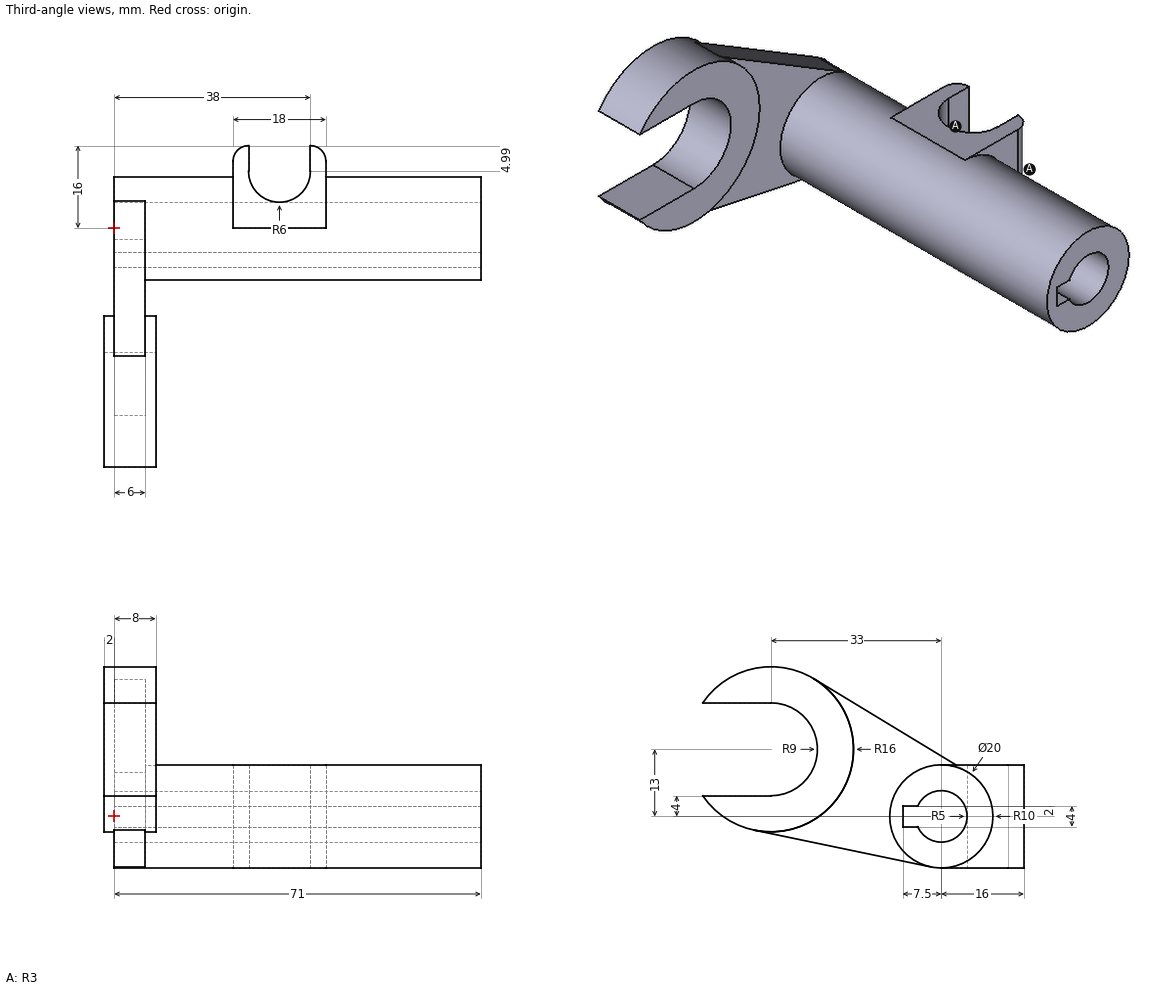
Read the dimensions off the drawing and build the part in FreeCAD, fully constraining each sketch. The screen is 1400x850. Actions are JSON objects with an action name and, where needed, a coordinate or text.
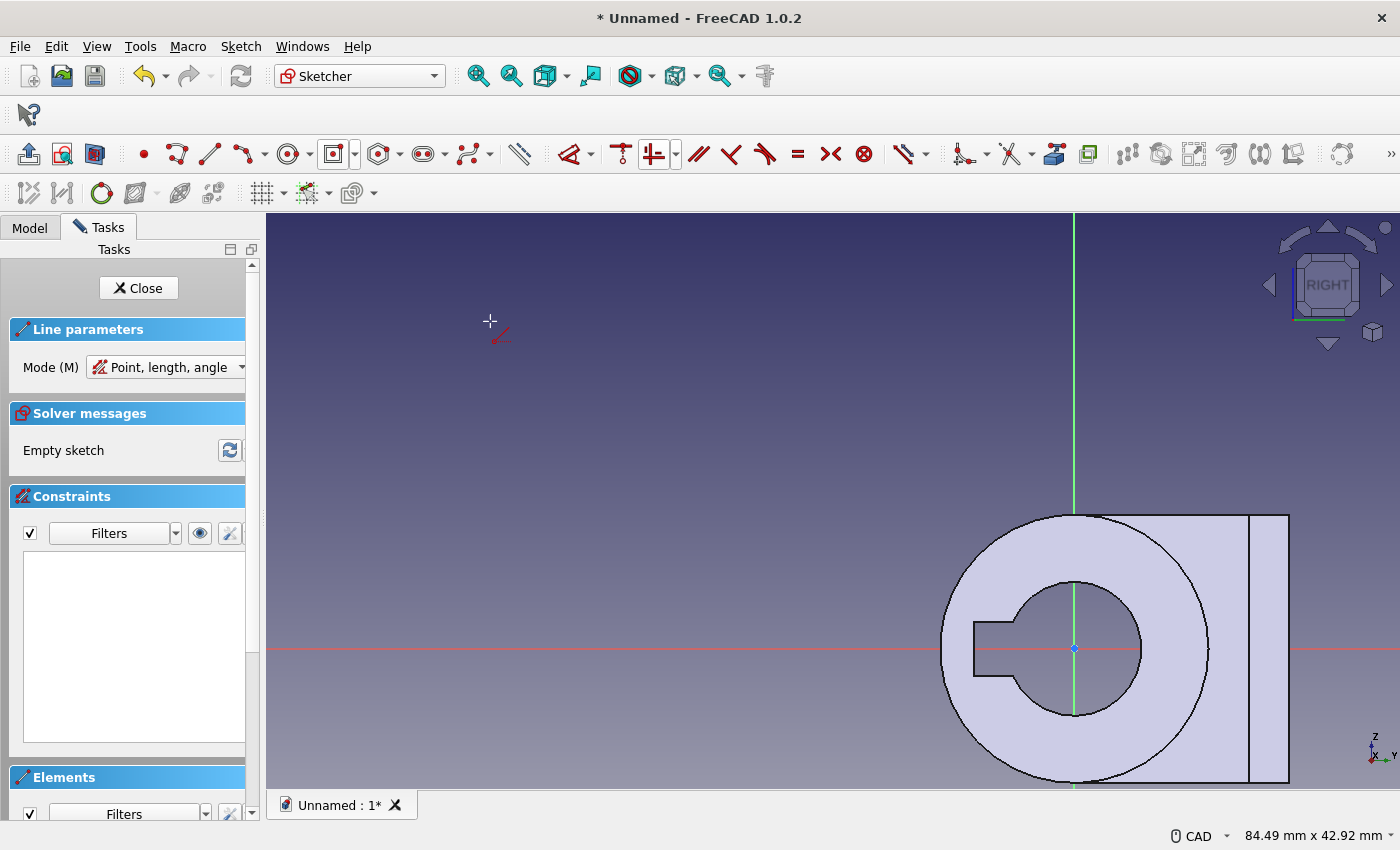
{"action": "left_click", "coordinate": [631, 354]}
{"action": "left_click", "coordinate": [454, 354]}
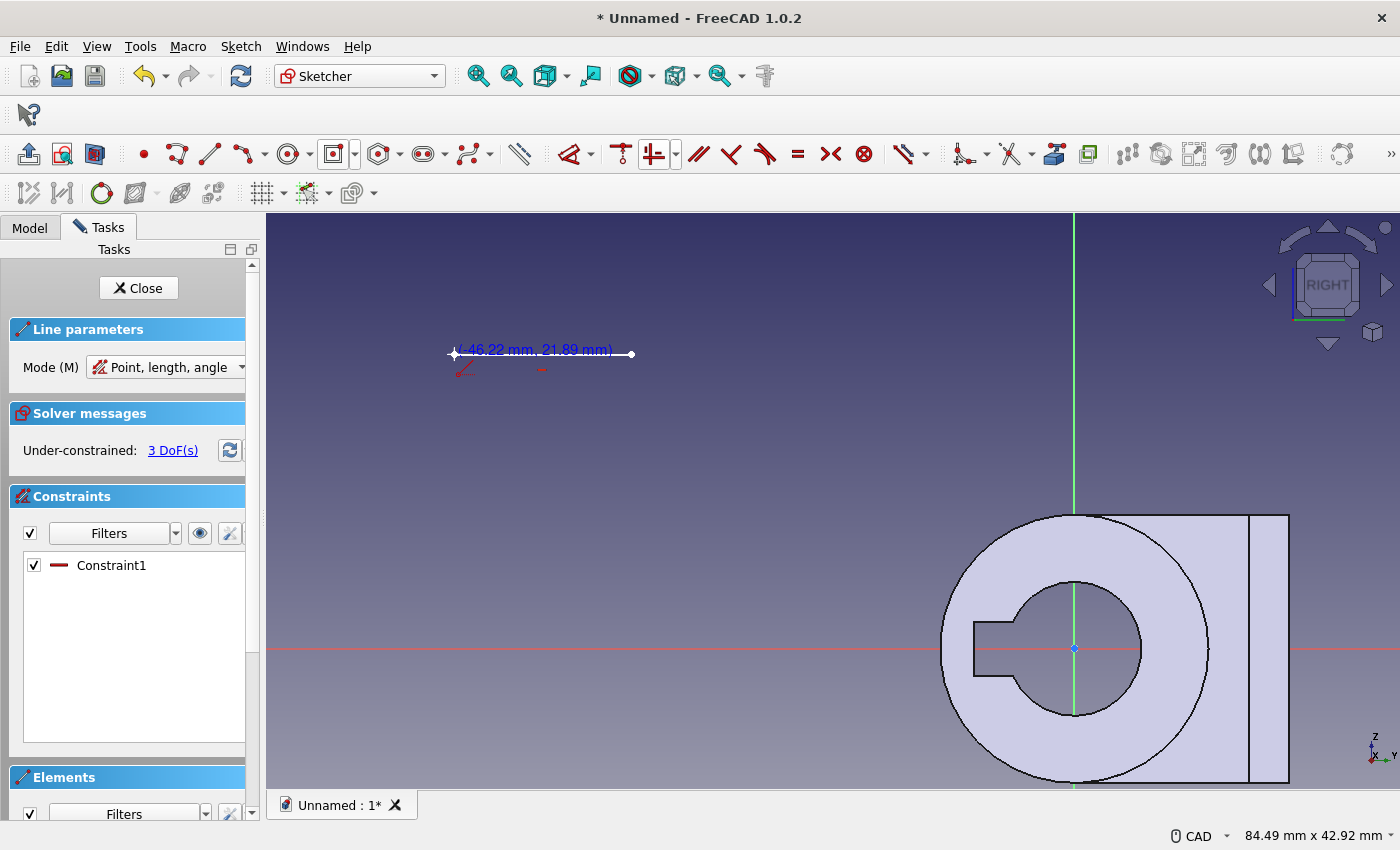
{"action": "left_click", "coordinate": [454, 595]}
{"action": "left_click", "coordinate": [631, 595]}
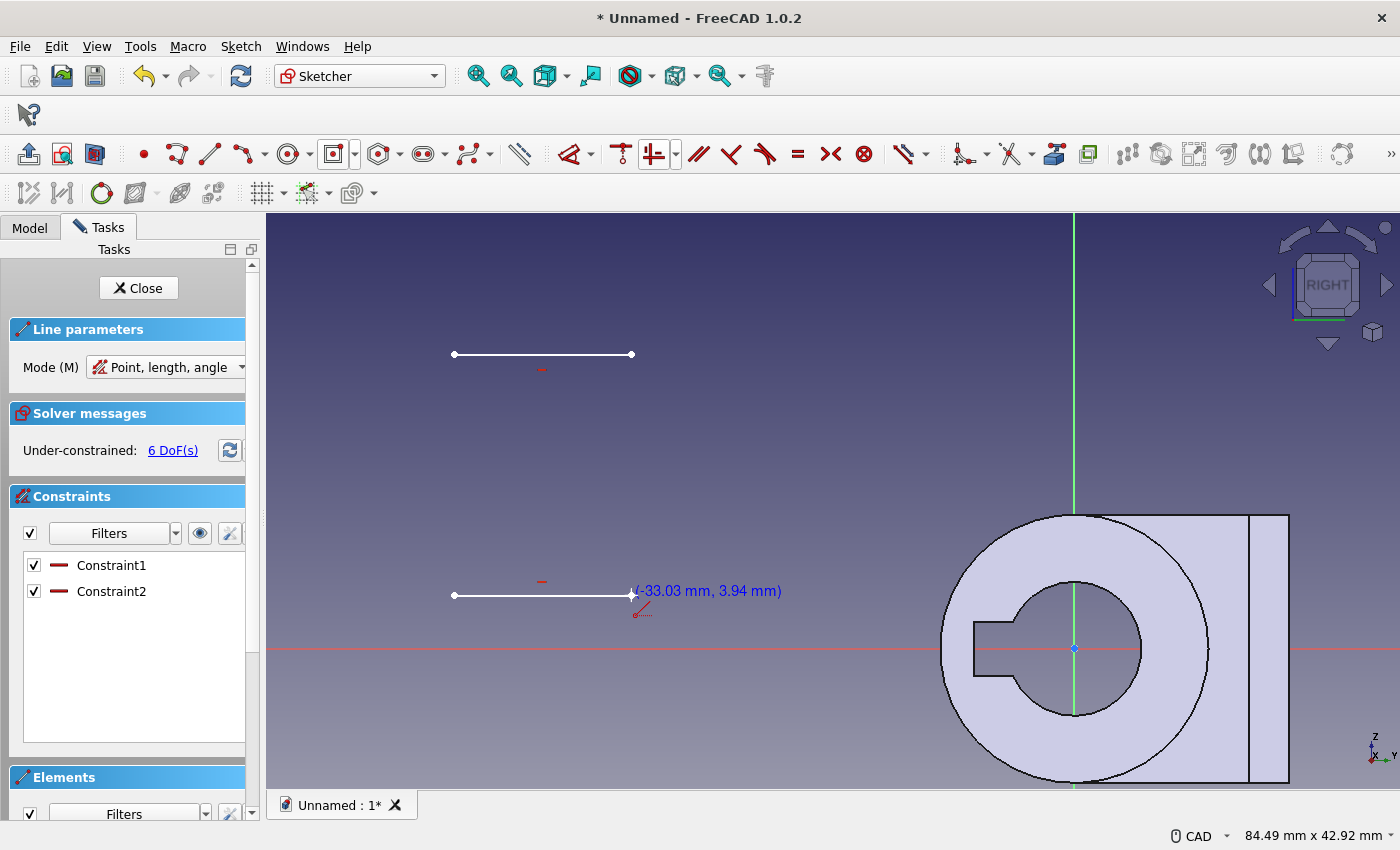
{"action": "key", "text": "g 3 a"}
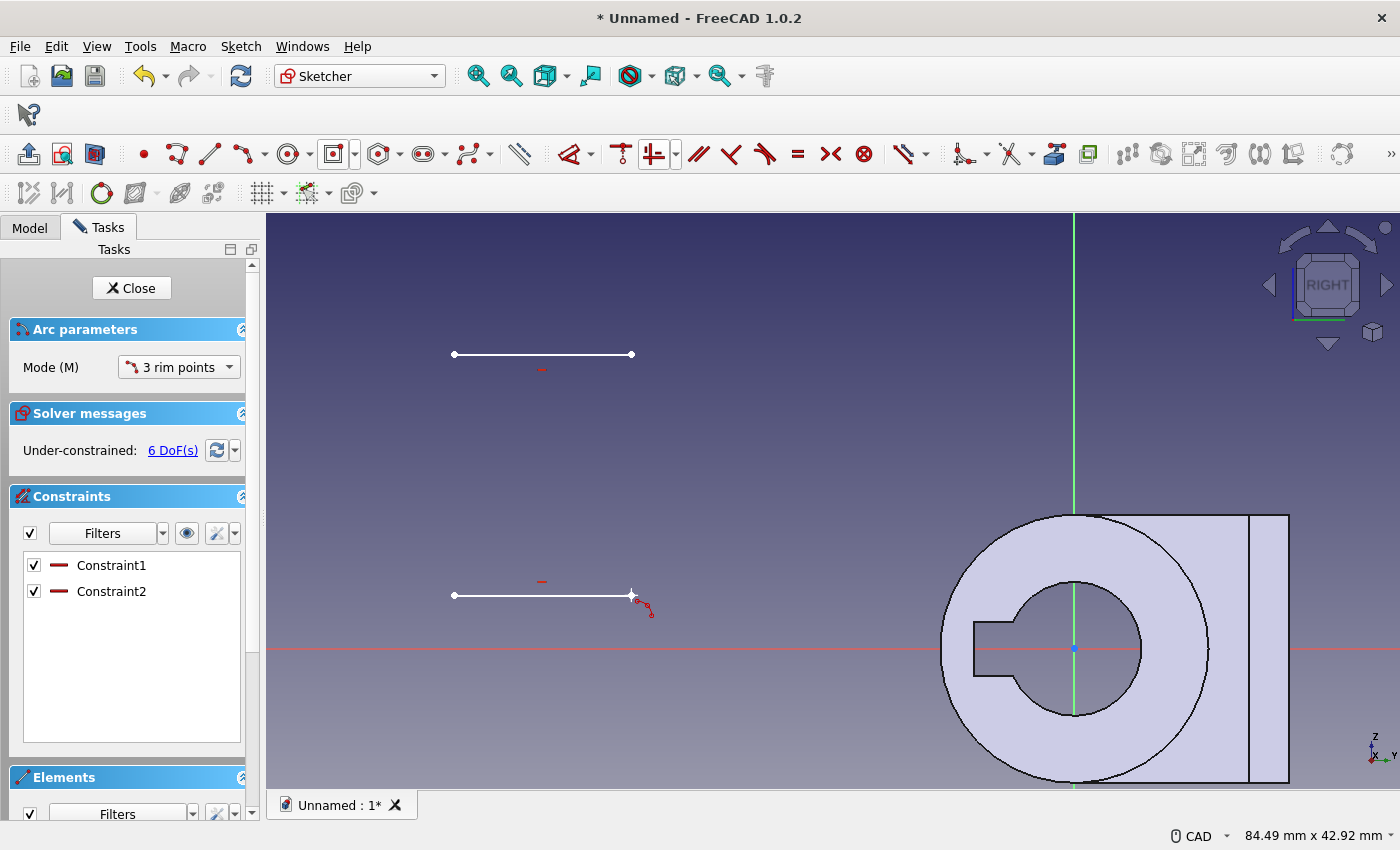
{"action": "left_click", "coordinate": [454, 355]}
{"action": "left_click", "coordinate": [454, 596]}
{"action": "left_click", "coordinate": [846, 474]}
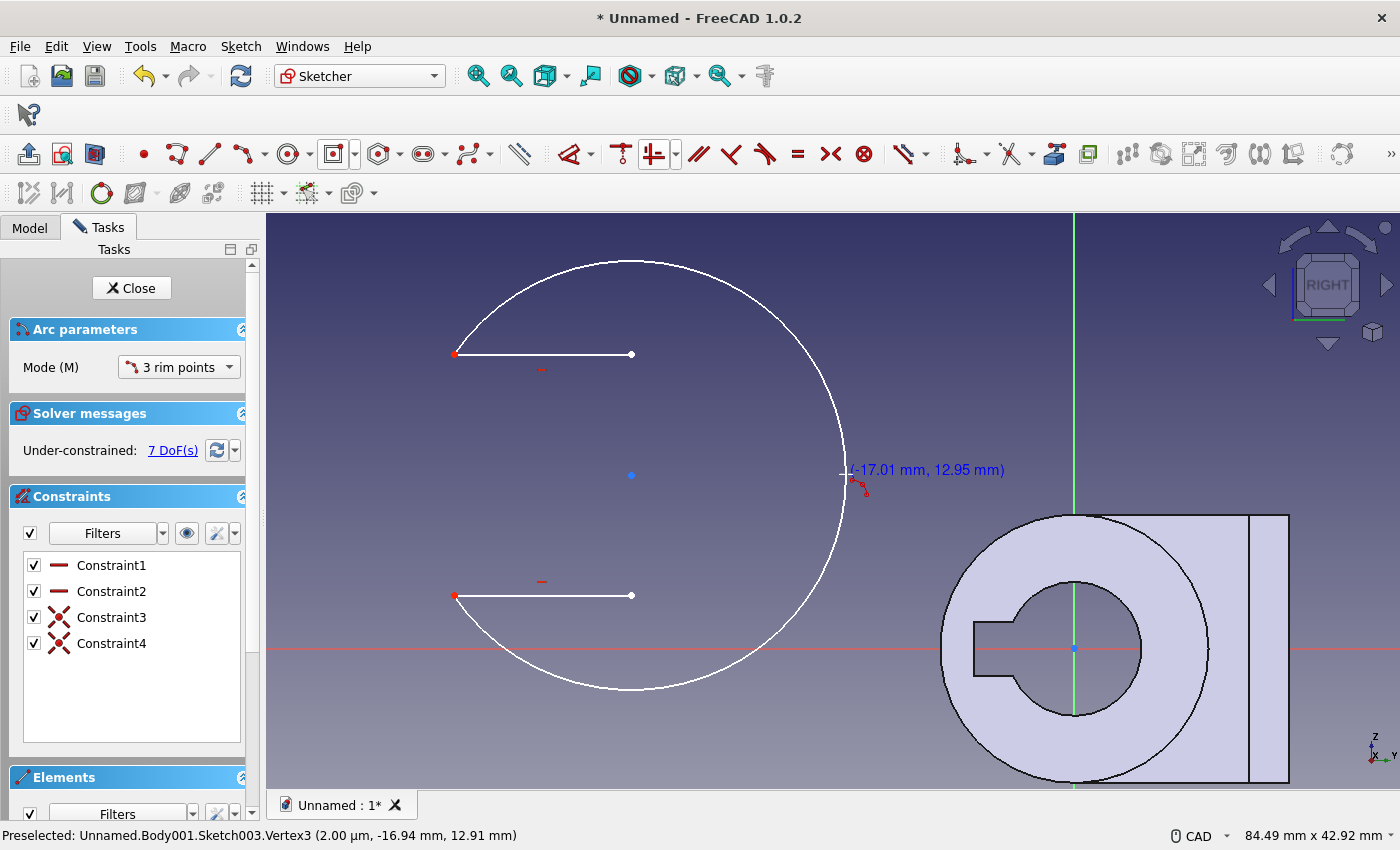
{"action": "left_click", "coordinate": [631, 596]}
{"action": "left_click", "coordinate": [631, 355]}
{"action": "left_click", "coordinate": [752, 474]}
{"action": "key", "text": "Escape"}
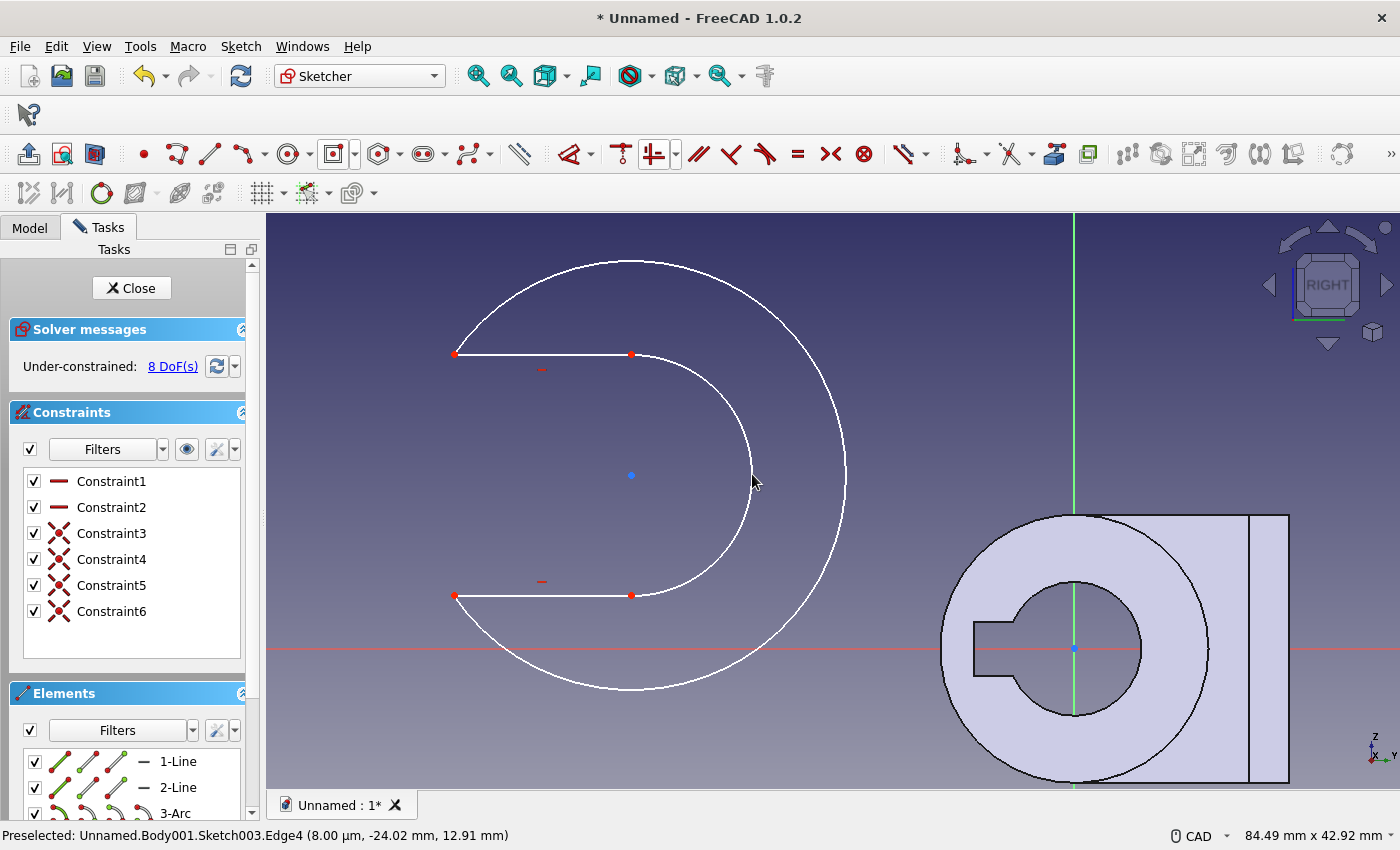
{"action": "left_click", "coordinate": [578, 355]}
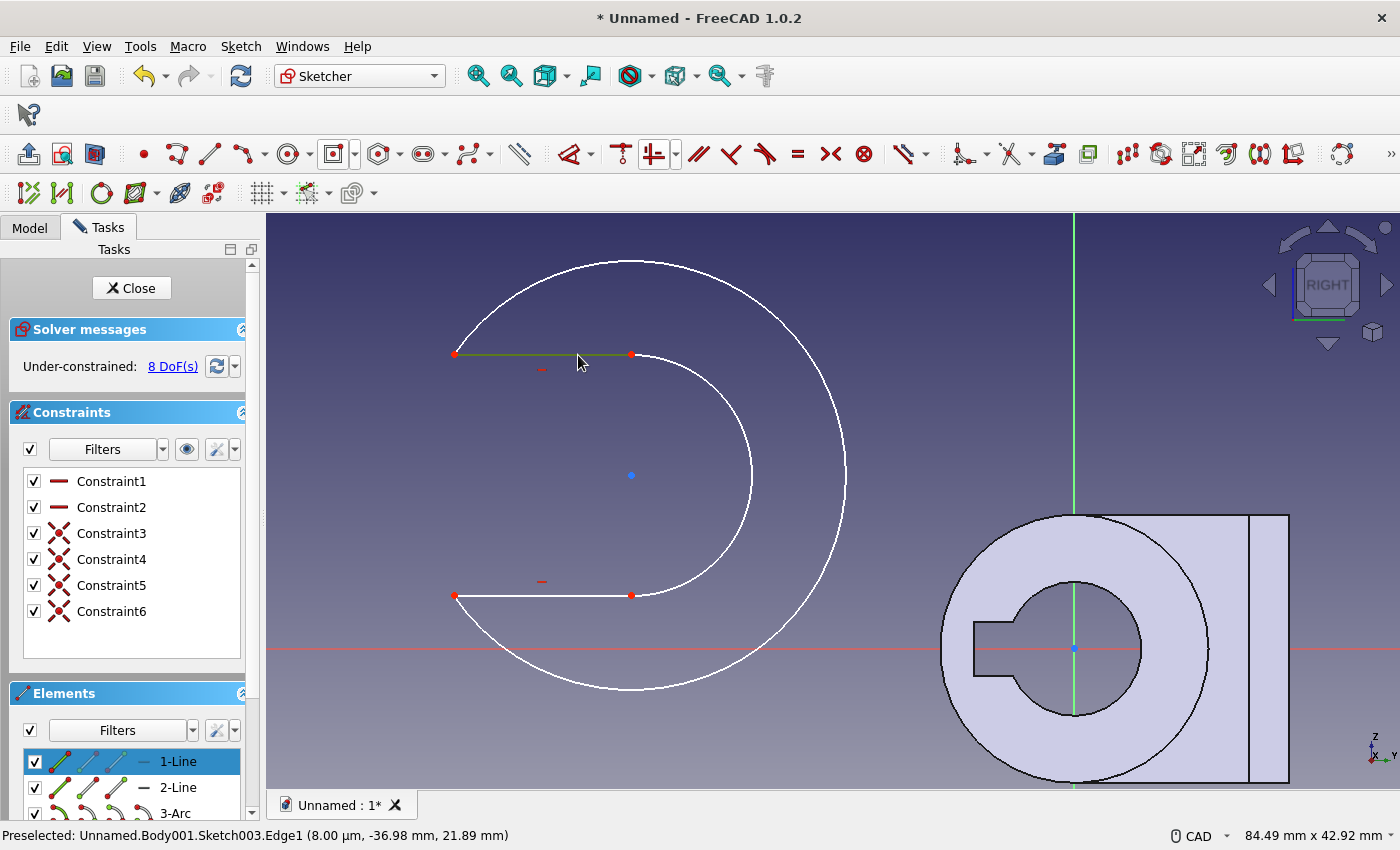
{"action": "left_click", "coordinate": [729, 546]}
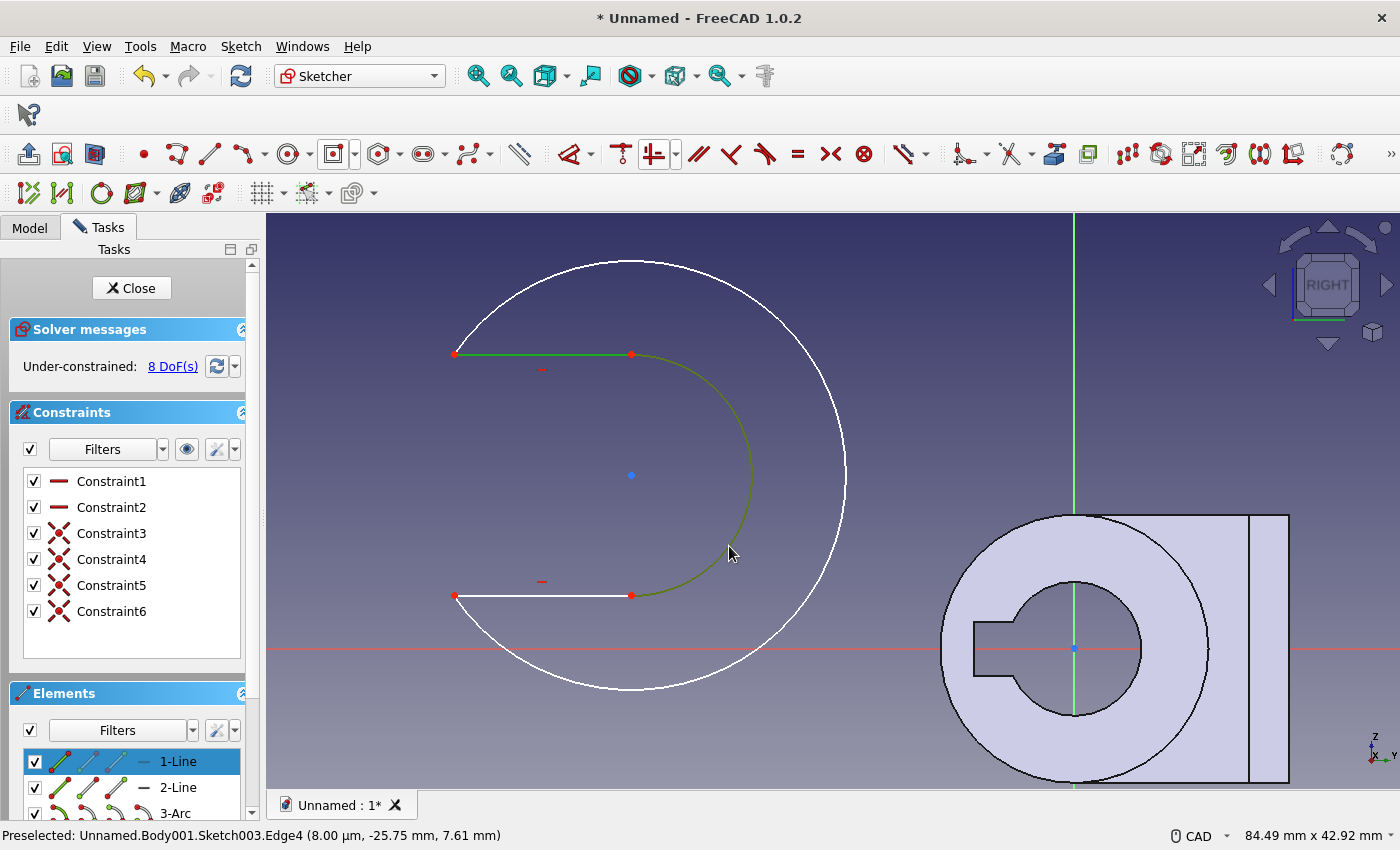
{"action": "left_click", "coordinate": [765, 154]}